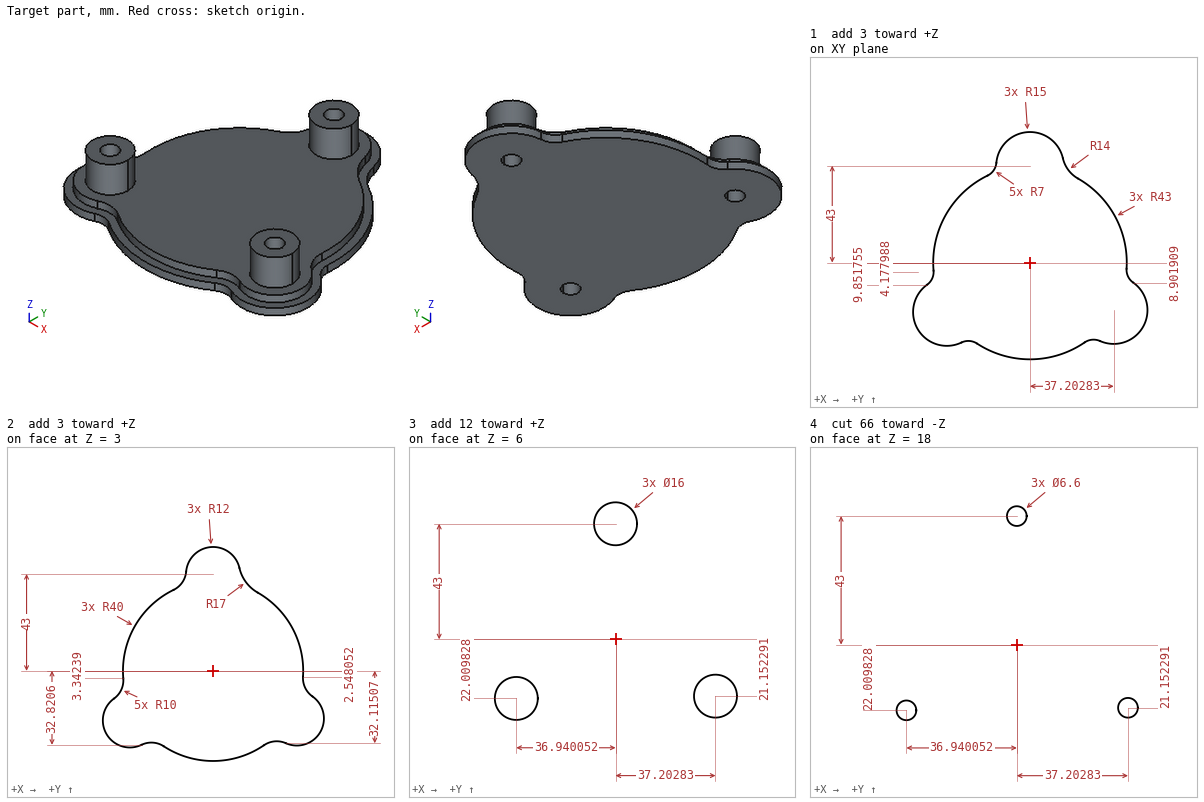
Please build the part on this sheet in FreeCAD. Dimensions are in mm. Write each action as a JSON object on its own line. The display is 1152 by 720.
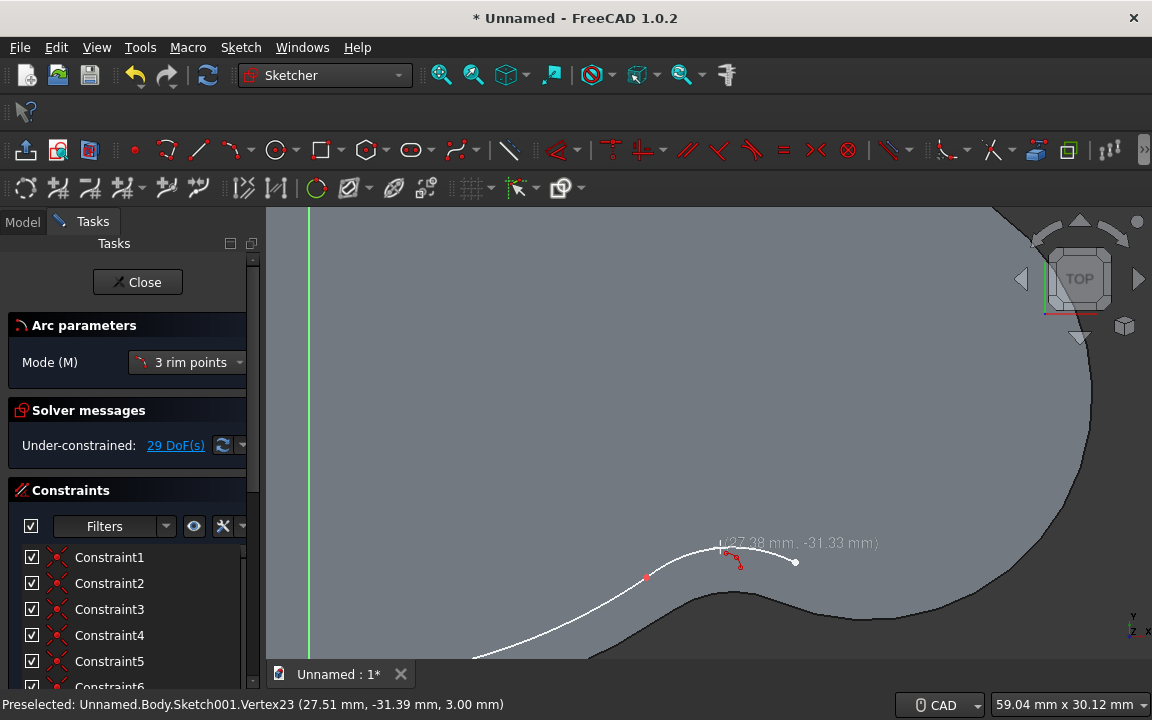
{"action": "scroll", "coordinate": [724, 551], "scroll_direction": "down", "scroll_amount": 8}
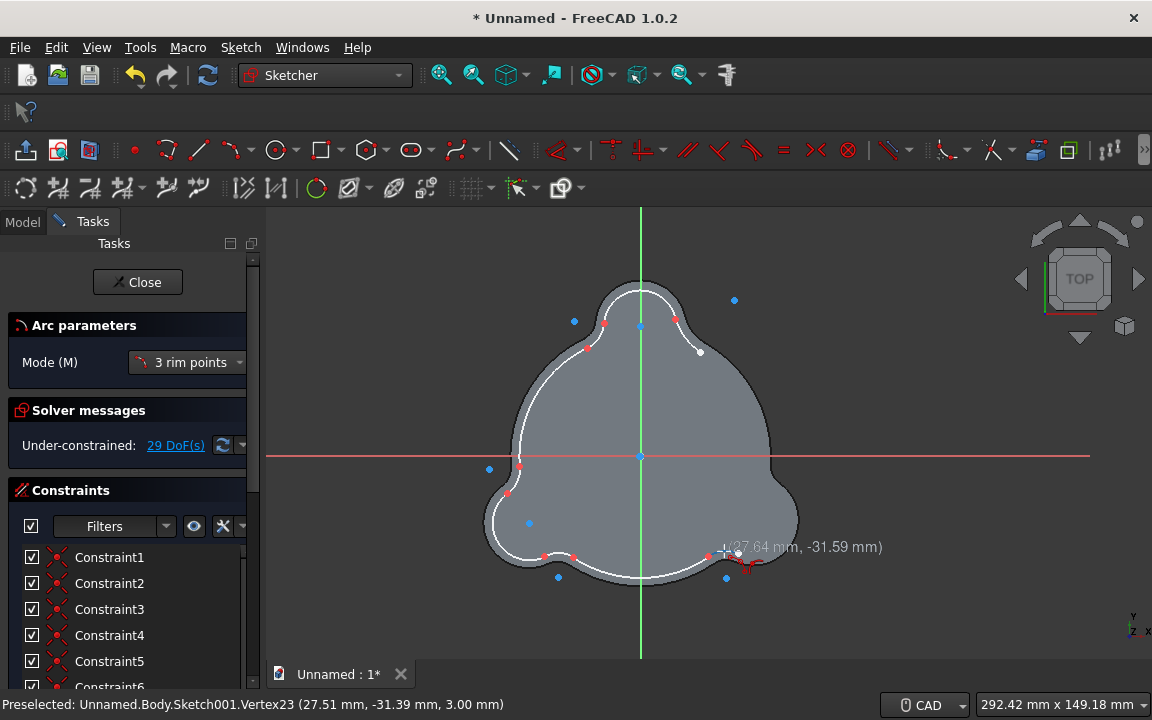
{"action": "left_click", "coordinate": [739, 554]}
{"action": "left_click", "coordinate": [774, 490]}
{"action": "left_click", "coordinate": [785, 538]}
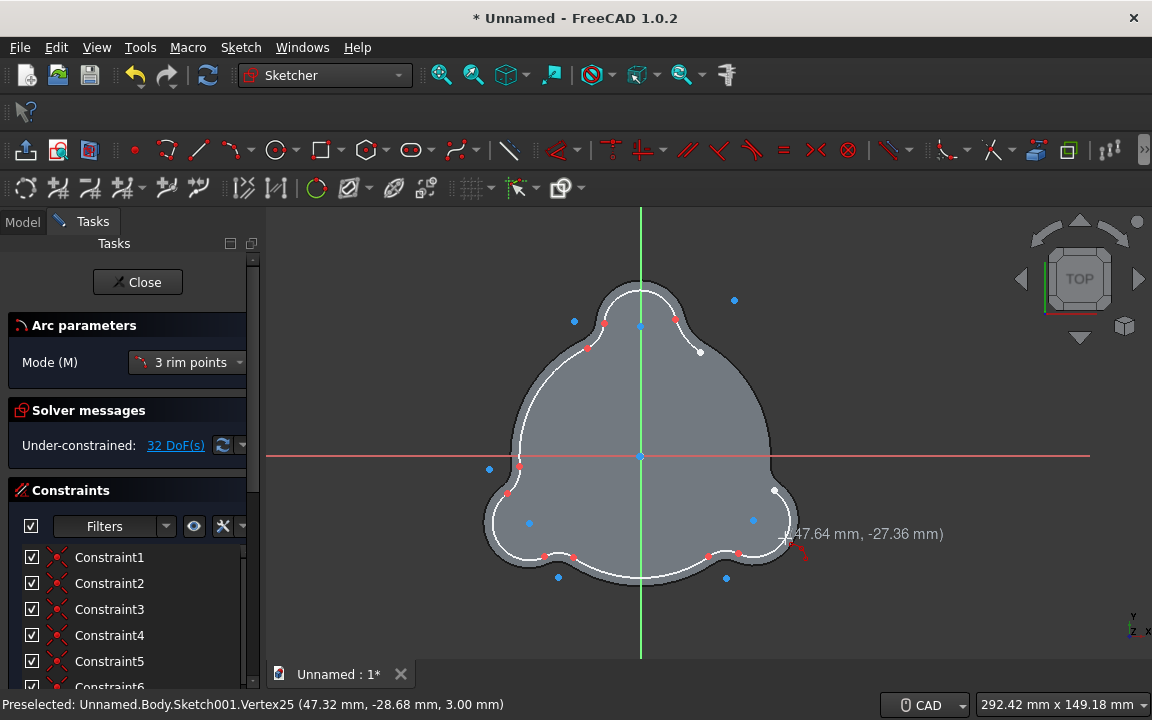
{"action": "left_click", "coordinate": [774, 491]}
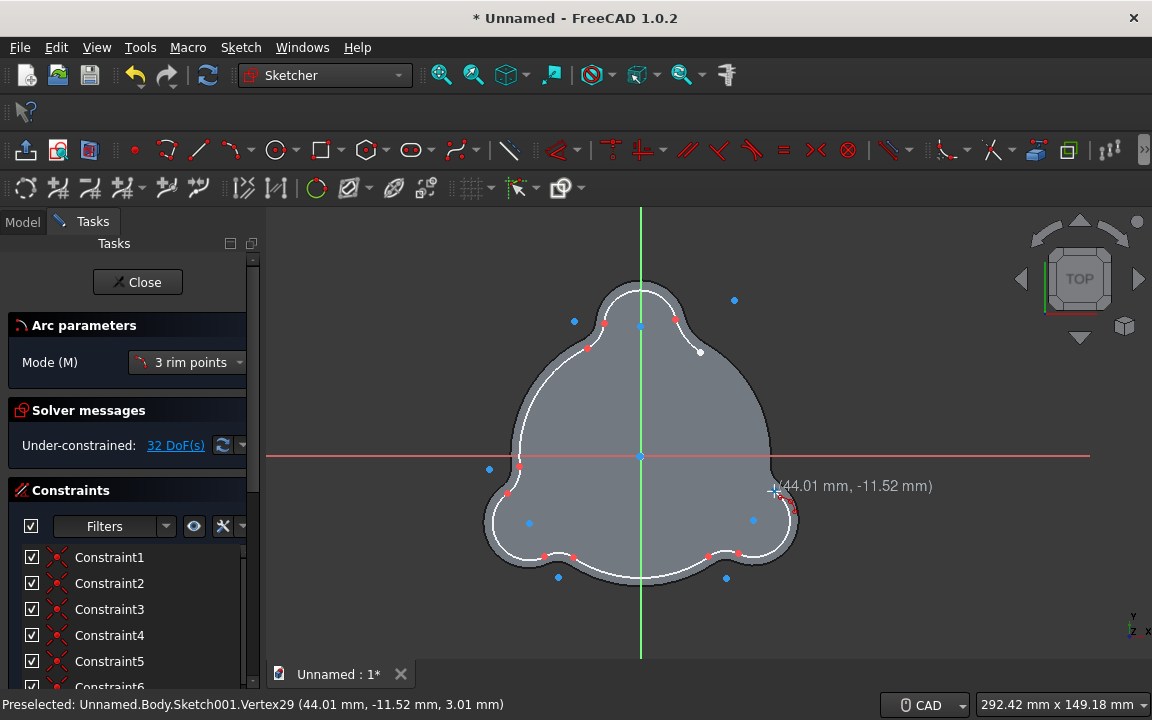
{"action": "scroll", "coordinate": [762, 464], "scroll_direction": "up", "scroll_amount": 4}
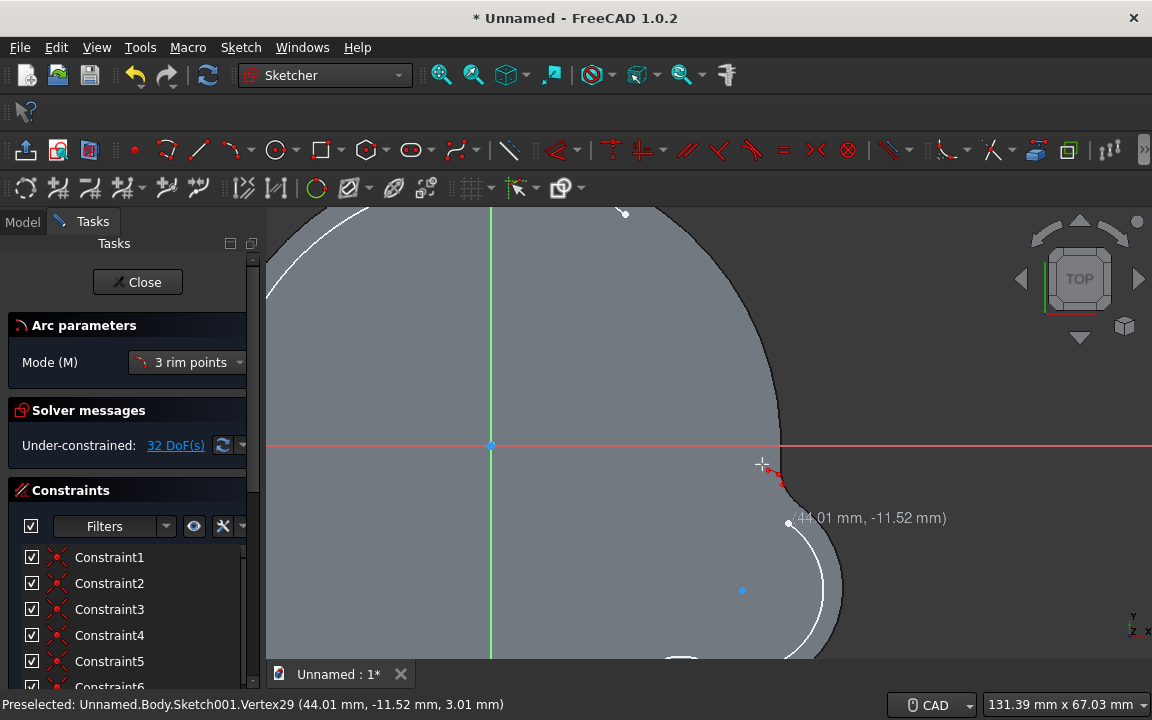
{"action": "left_click", "coordinate": [760, 463]}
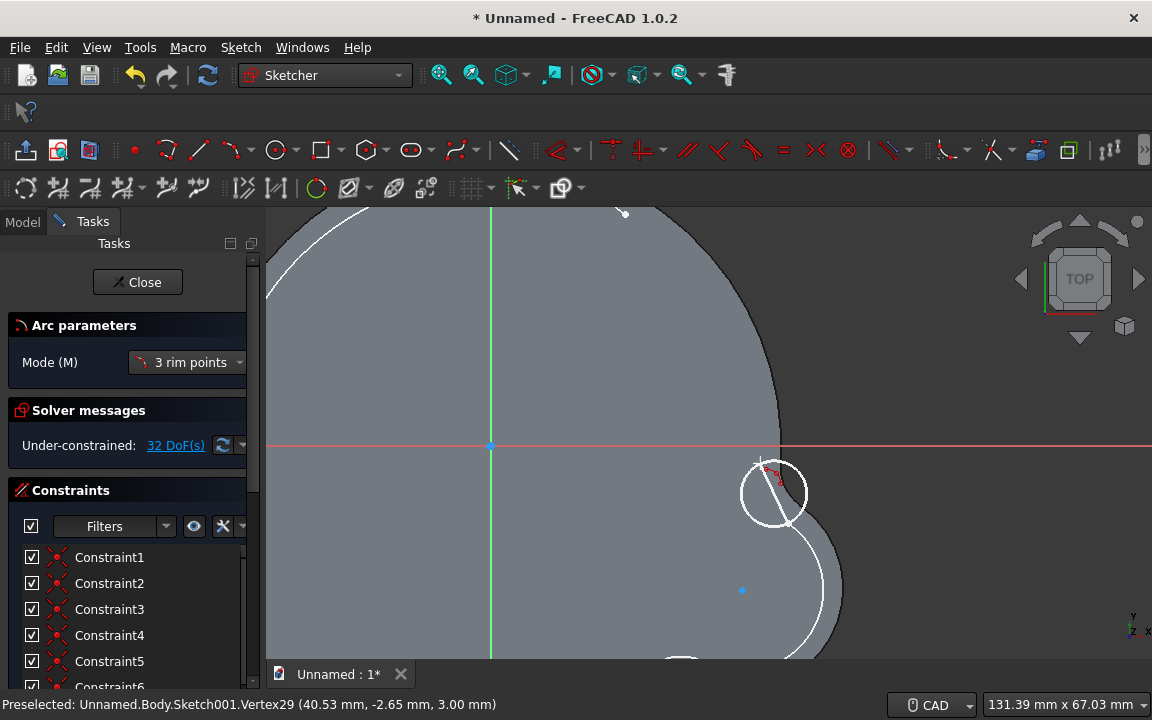
{"action": "scroll", "coordinate": [767, 496], "scroll_direction": "up", "scroll_amount": 4}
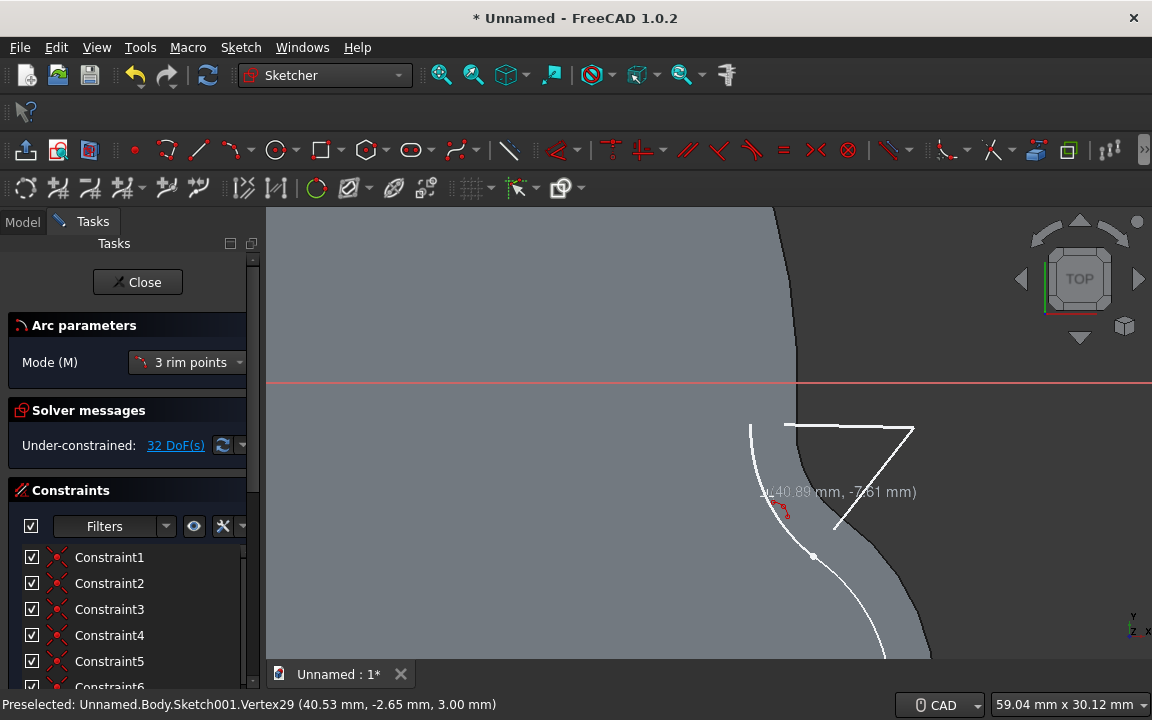
{"action": "left_click", "coordinate": [766, 496]}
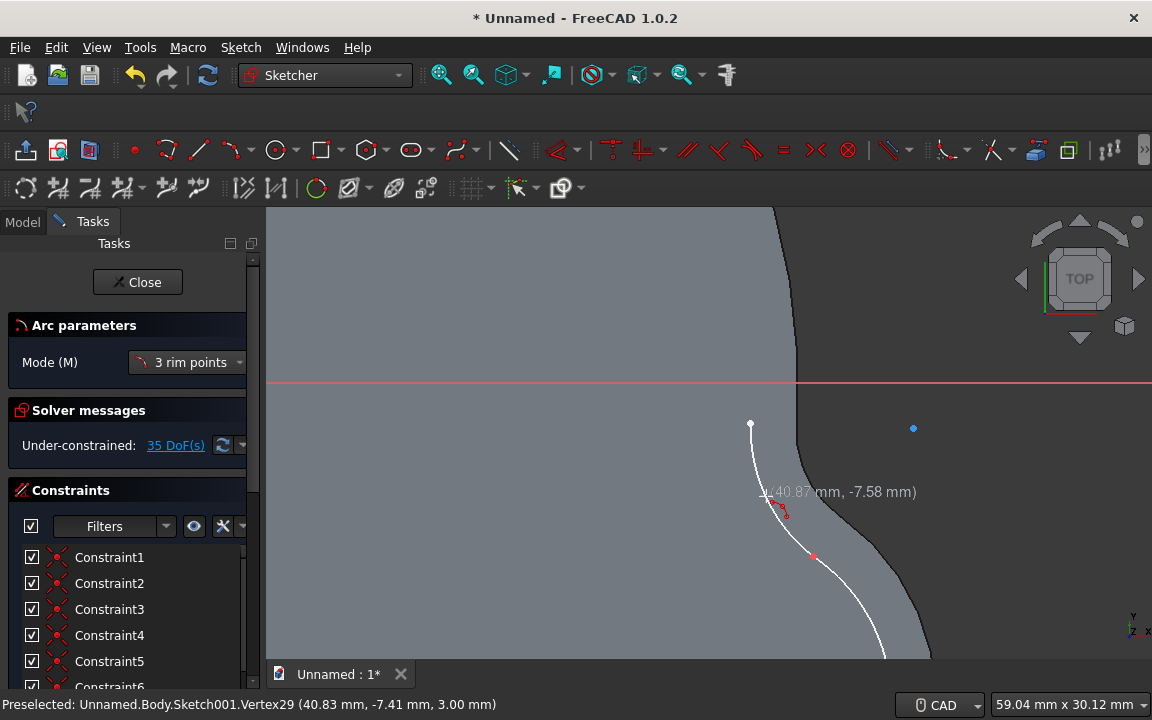
{"action": "left_click", "coordinate": [751, 424]}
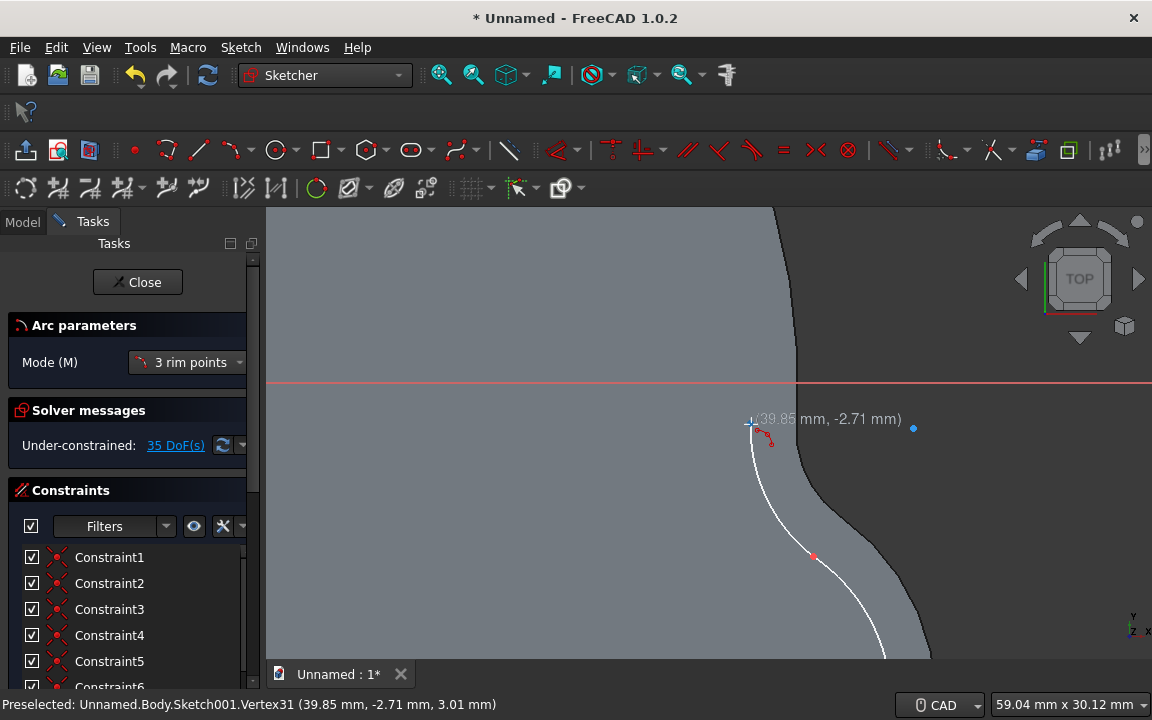
{"action": "scroll", "coordinate": [763, 474], "scroll_direction": "down", "scroll_amount": 8}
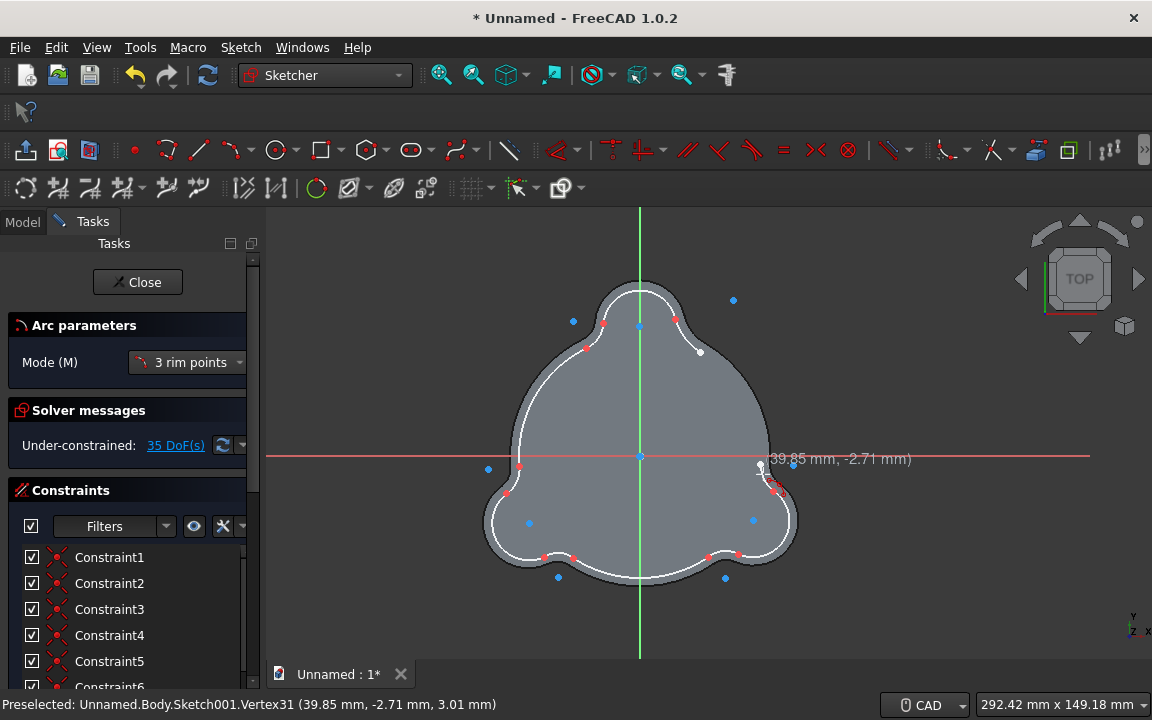
{"action": "left_click", "coordinate": [700, 352]}
{"action": "left_click", "coordinate": [747, 399]}
{"action": "key", "text": "Escape"}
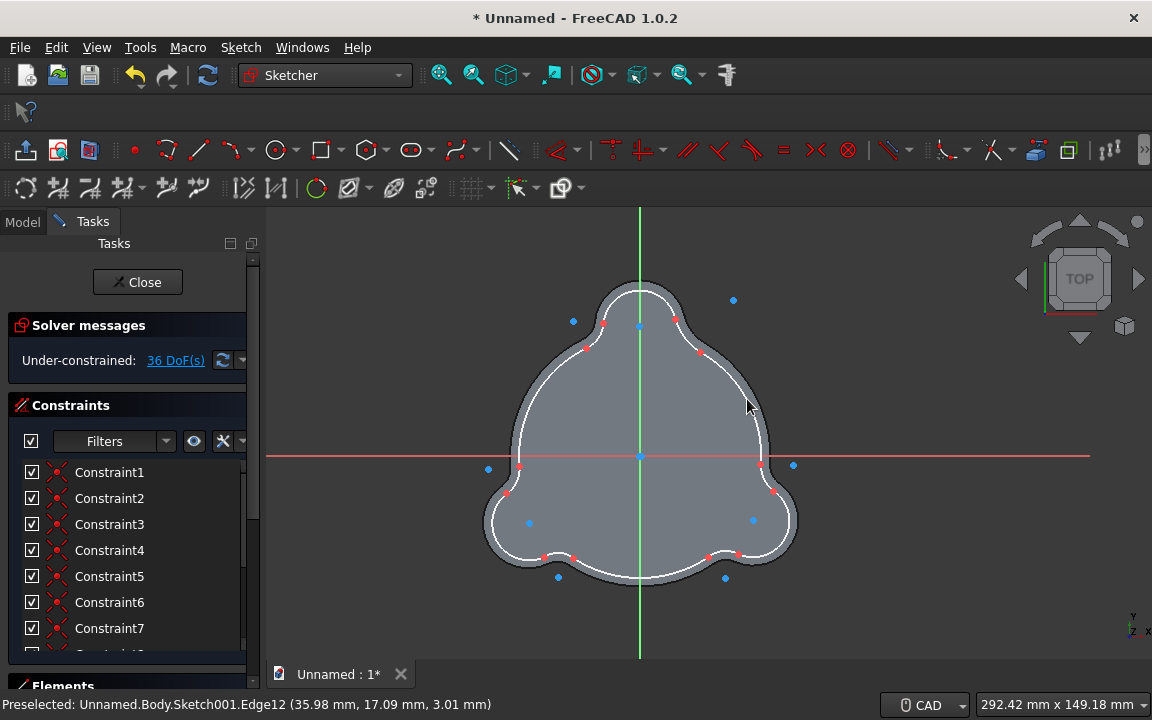
{"action": "left_click", "coordinate": [680, 331]}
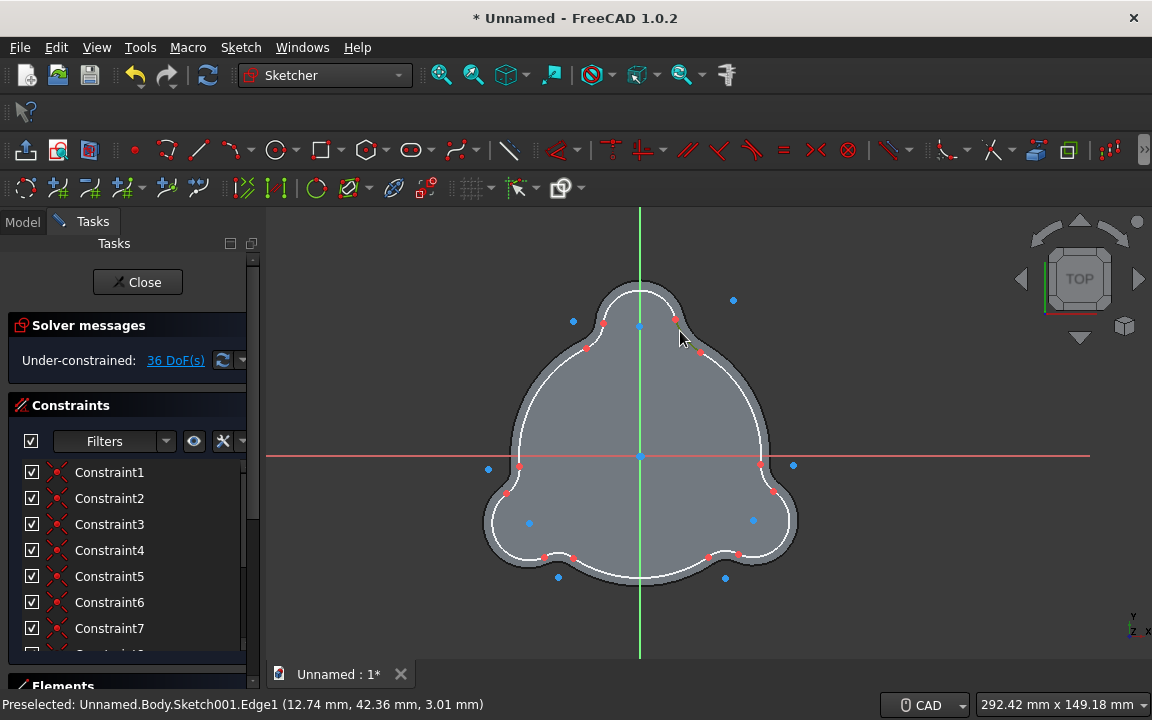
{"action": "left_click", "coordinate": [658, 295]}